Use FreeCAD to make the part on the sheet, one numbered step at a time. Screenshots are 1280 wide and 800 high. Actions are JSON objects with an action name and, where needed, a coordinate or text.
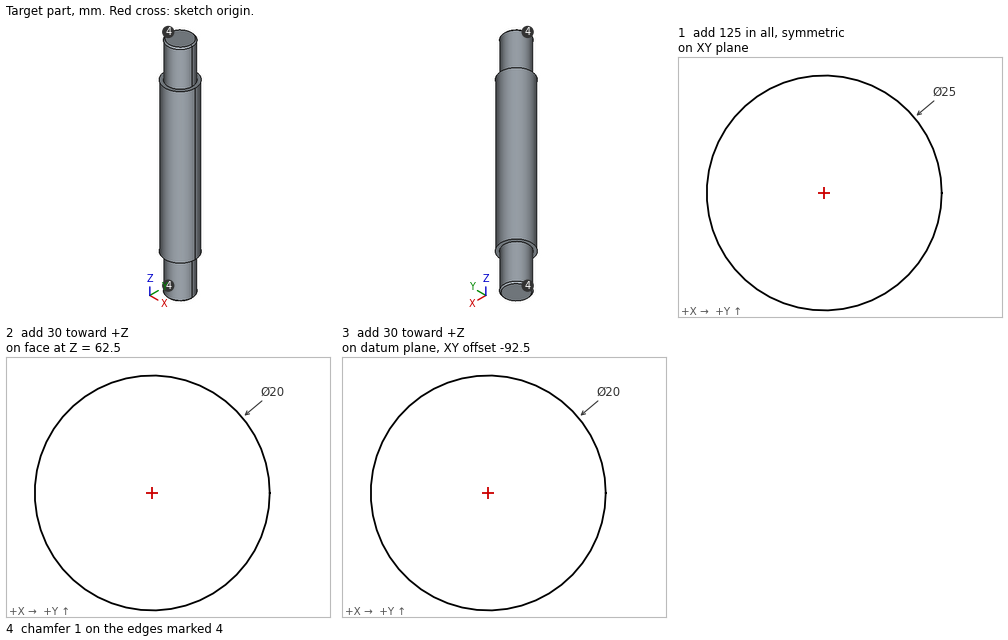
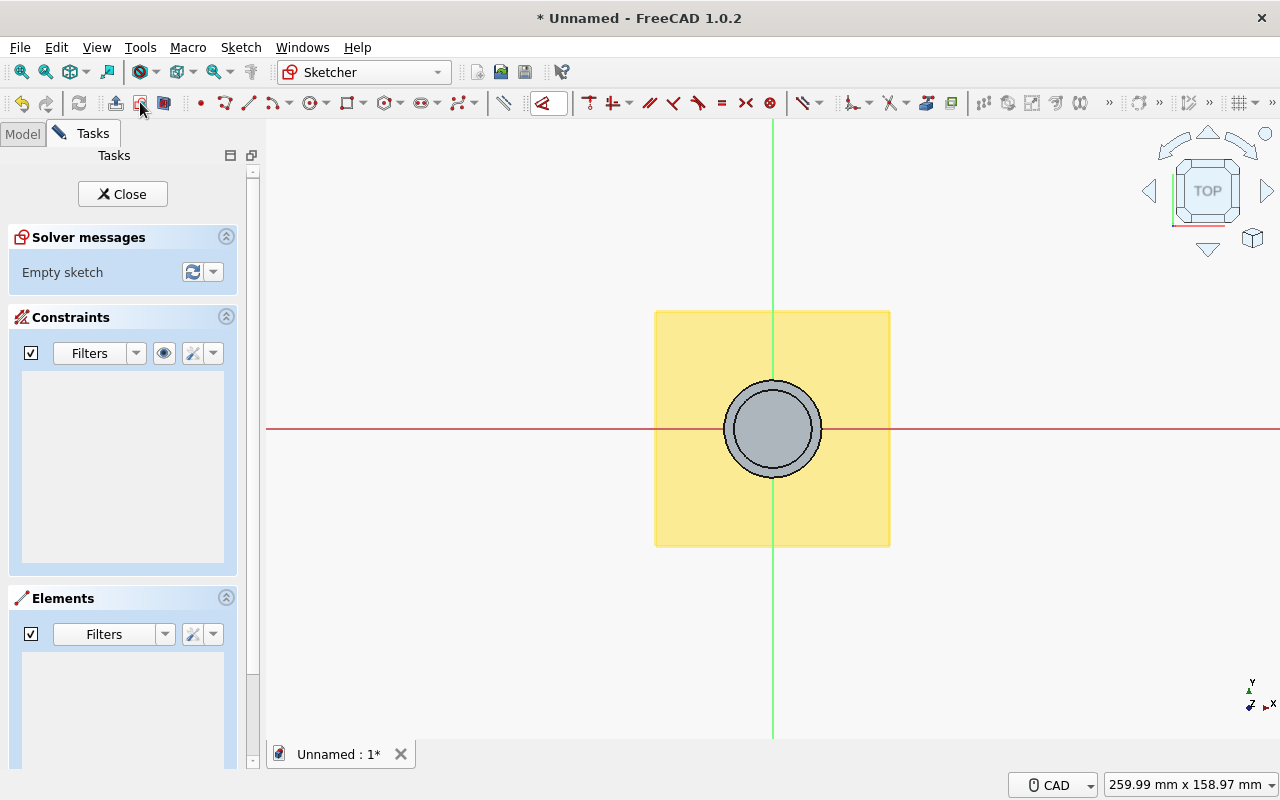
{"action": "key", "text": "q s"}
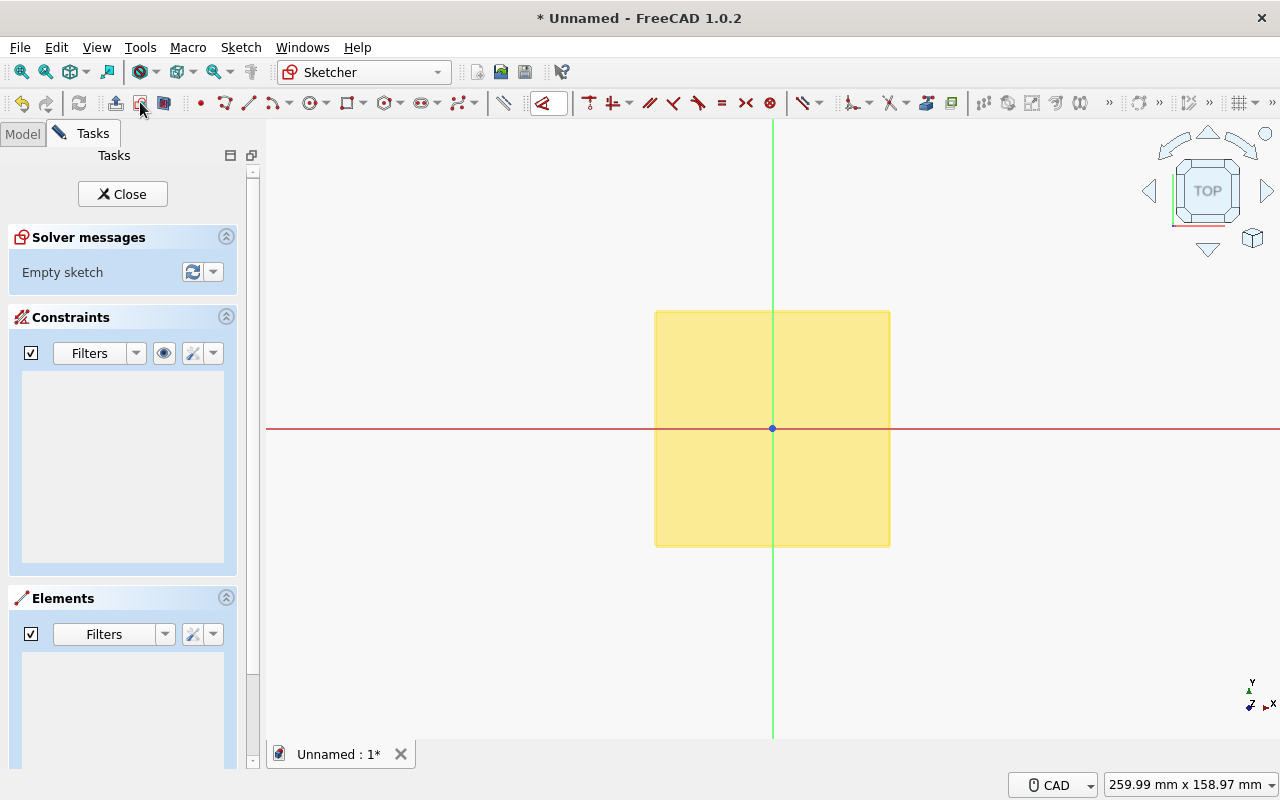
{"action": "scroll", "coordinate": [790, 429], "scroll_direction": "up", "scroll_amount": 8}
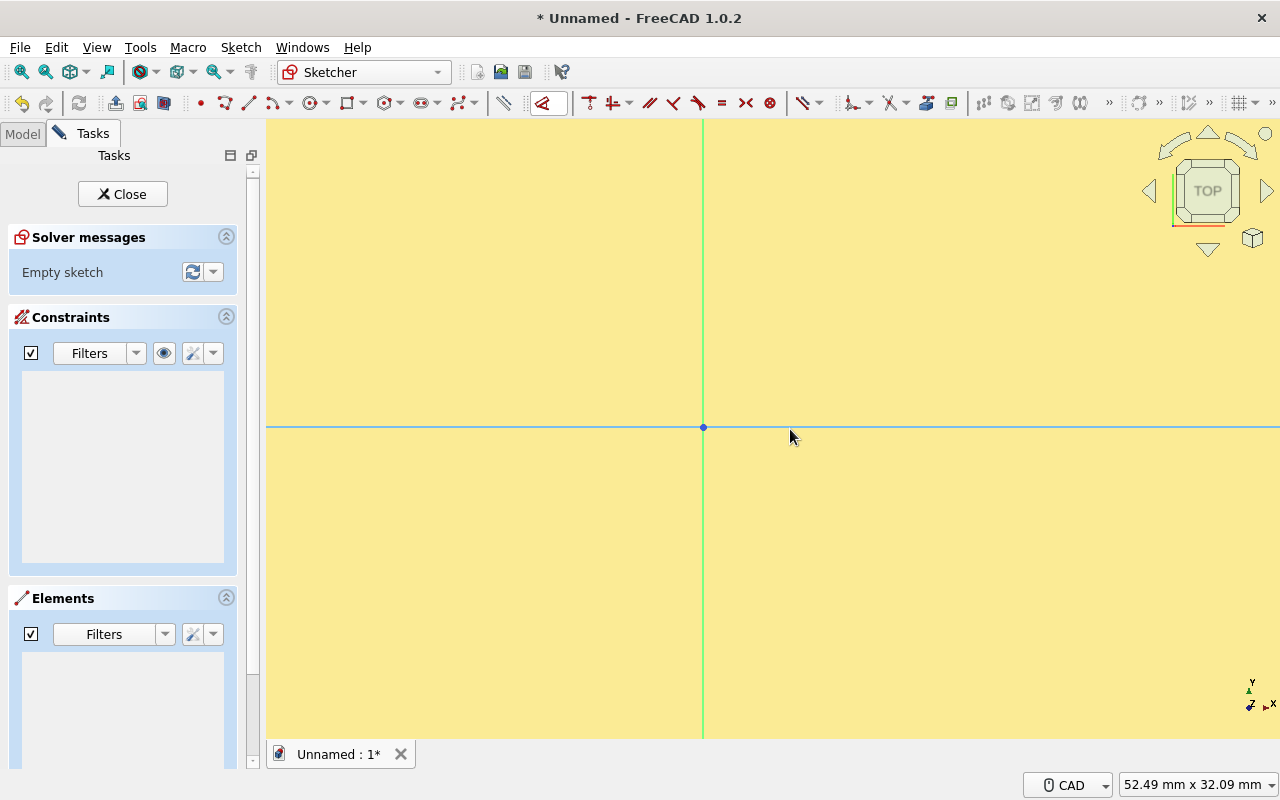
{"action": "left_click", "coordinate": [310, 104]}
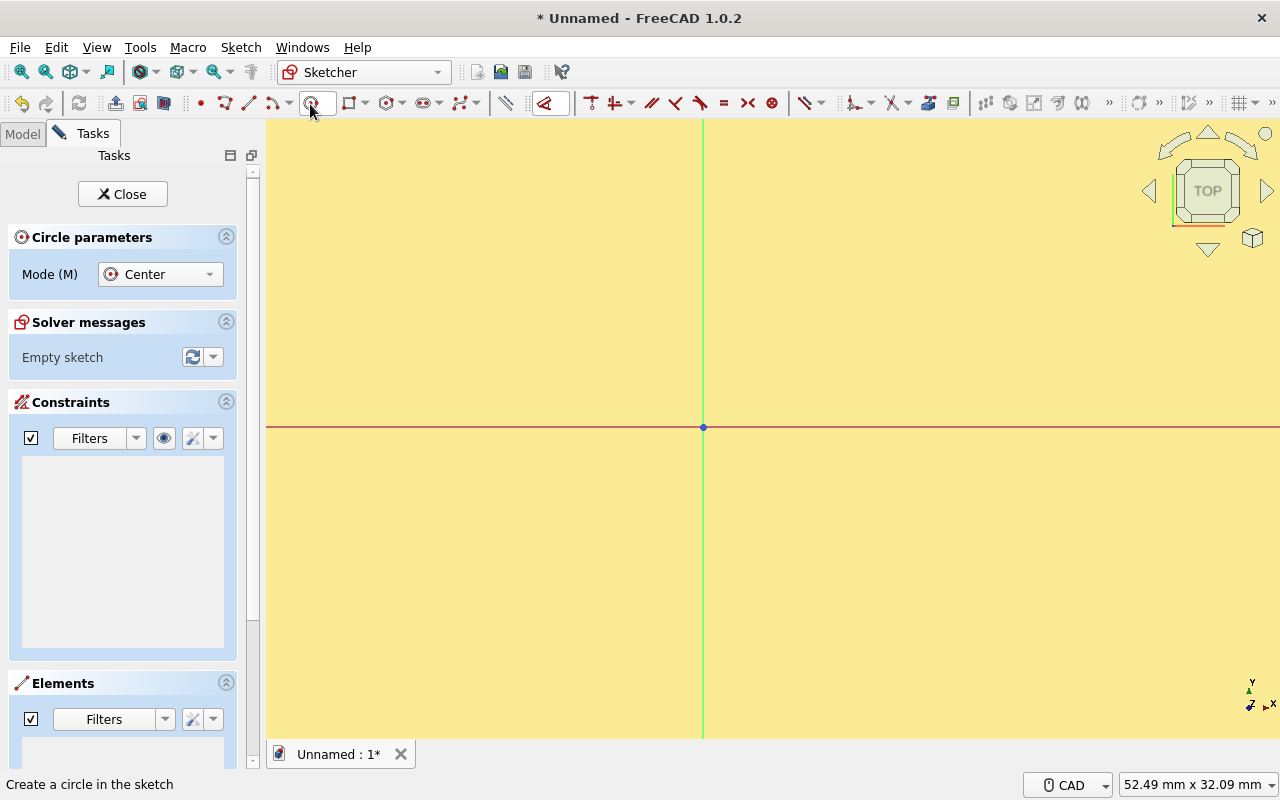
{"action": "left_click", "coordinate": [703, 427]}
{"action": "left_click", "coordinate": [840, 290]}
{"action": "key", "text": "Escape"}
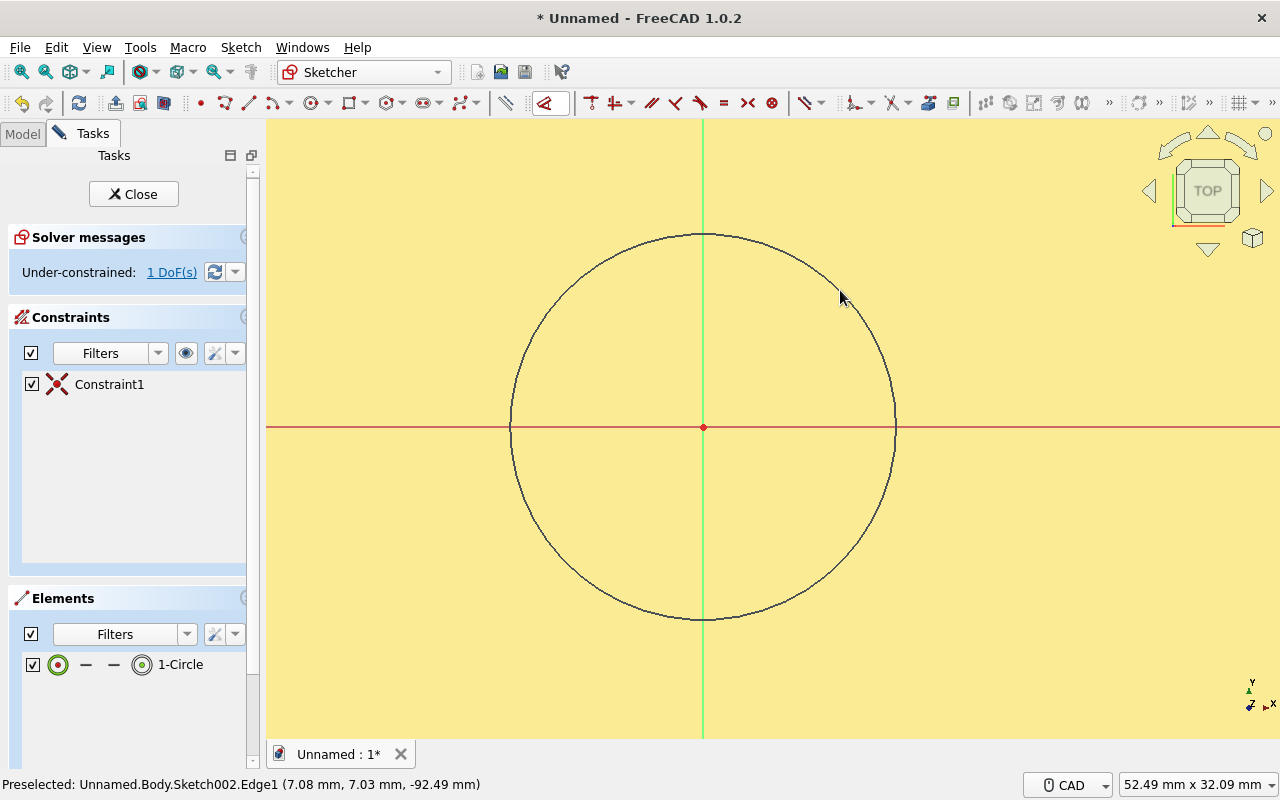
{"action": "left_click", "coordinate": [839, 290]}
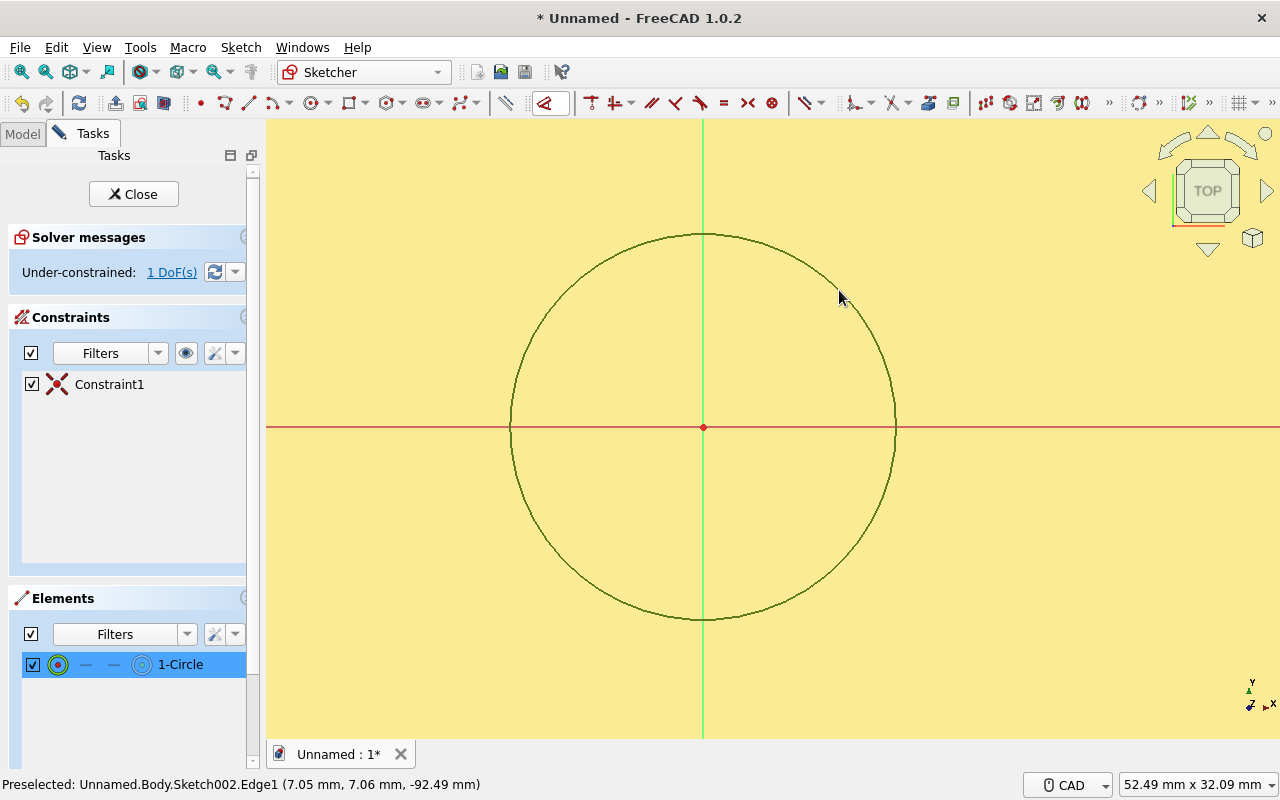
{"action": "left_click", "coordinate": [564, 104]}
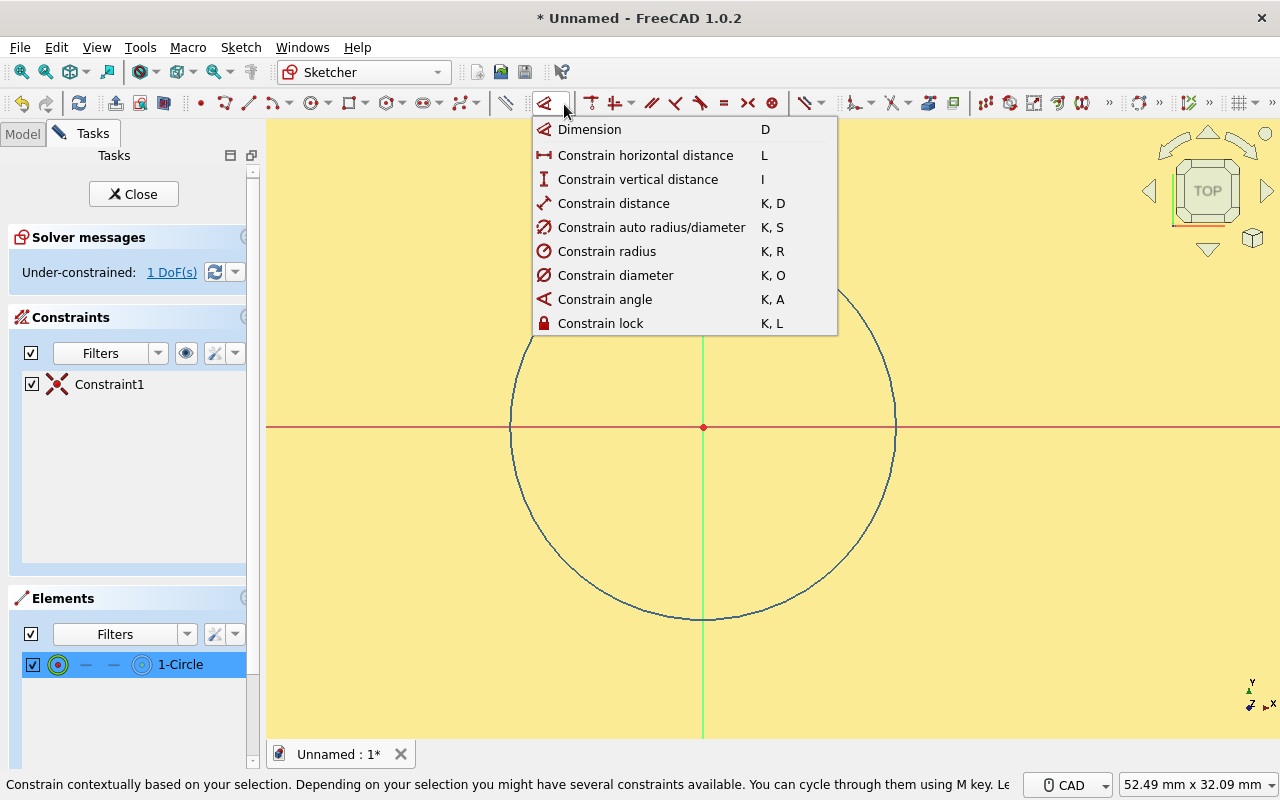
{"action": "left_click", "coordinate": [685, 275]}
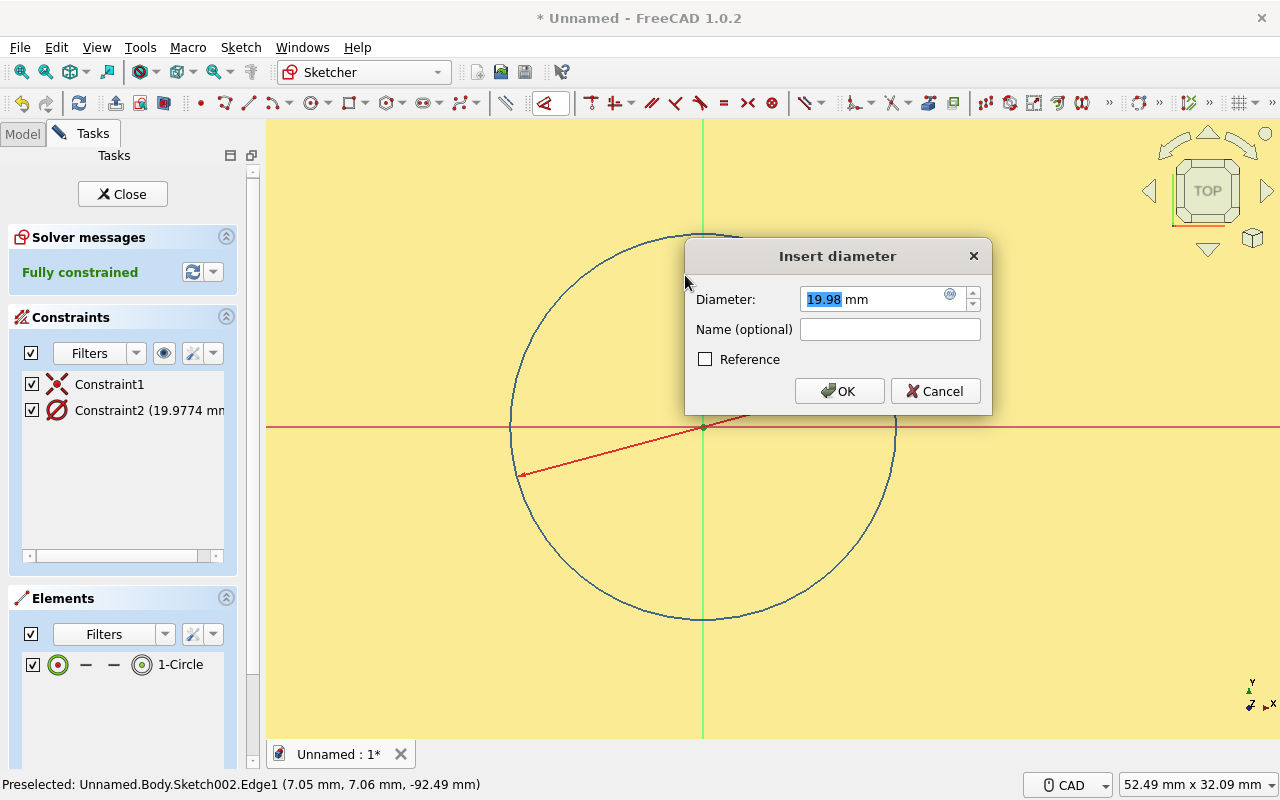
{"action": "type", "text": "20"}
{"action": "key", "text": "Return"}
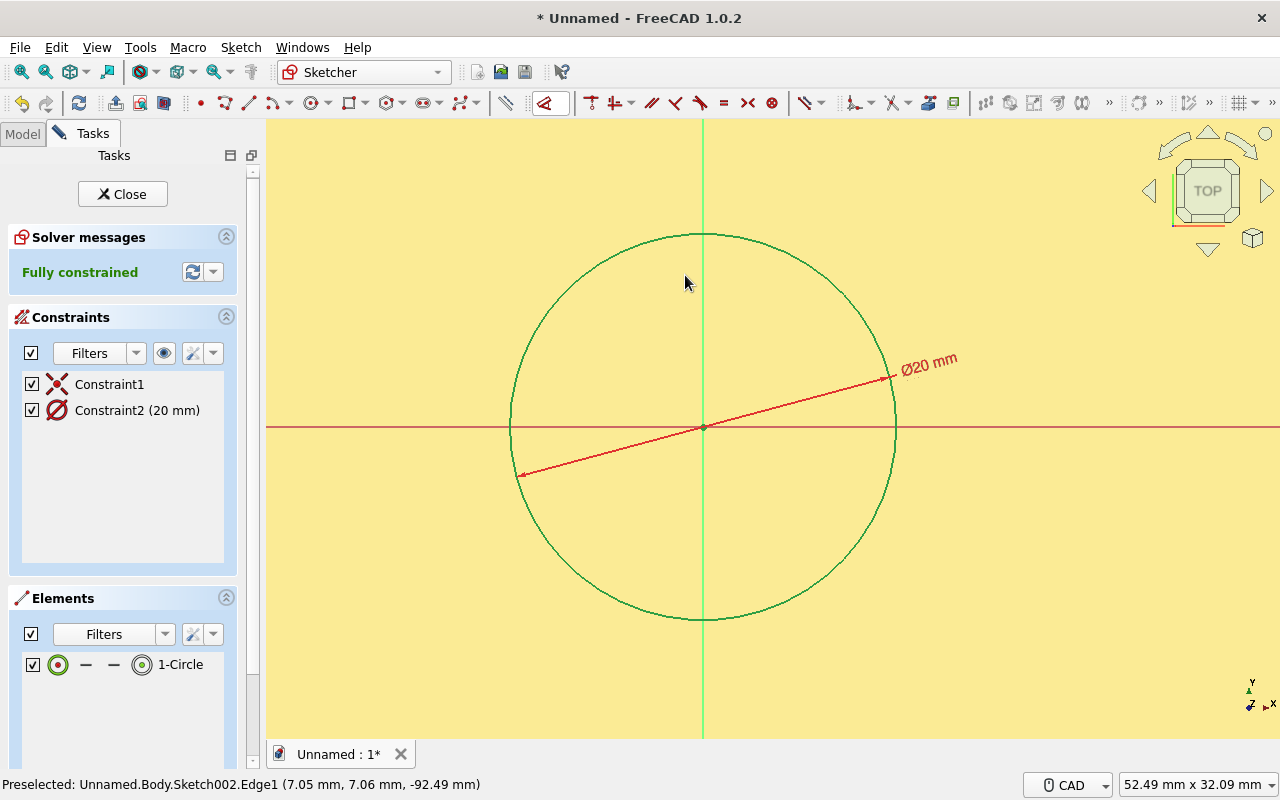
{"action": "left_click", "coordinate": [123, 194]}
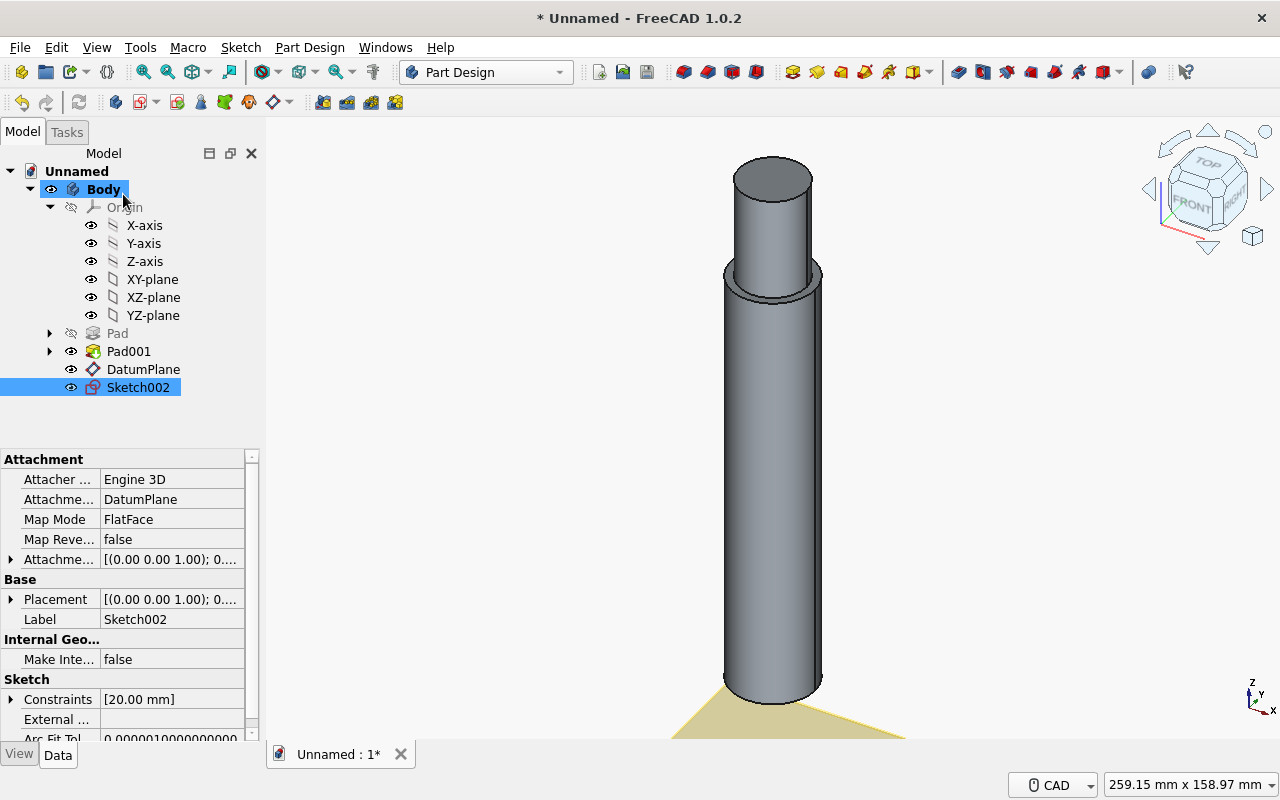
{"action": "left_click", "coordinate": [794, 72]}